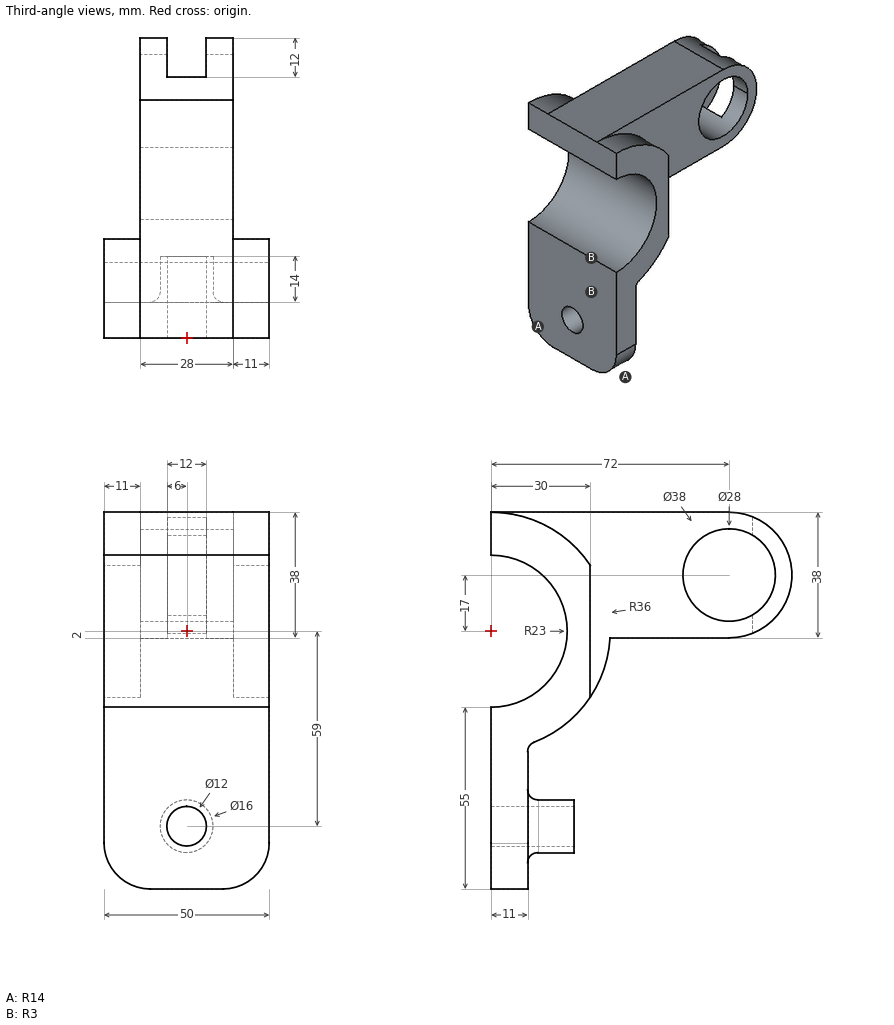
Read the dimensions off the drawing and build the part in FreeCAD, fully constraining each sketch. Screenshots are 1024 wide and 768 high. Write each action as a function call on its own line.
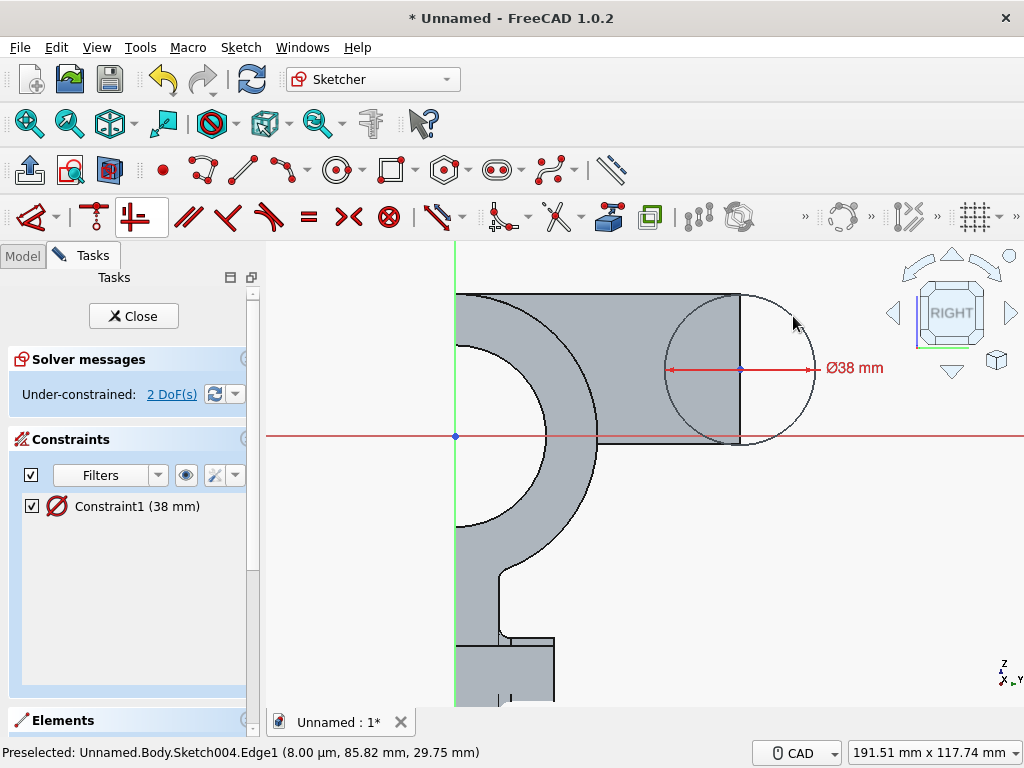
click(32, 218)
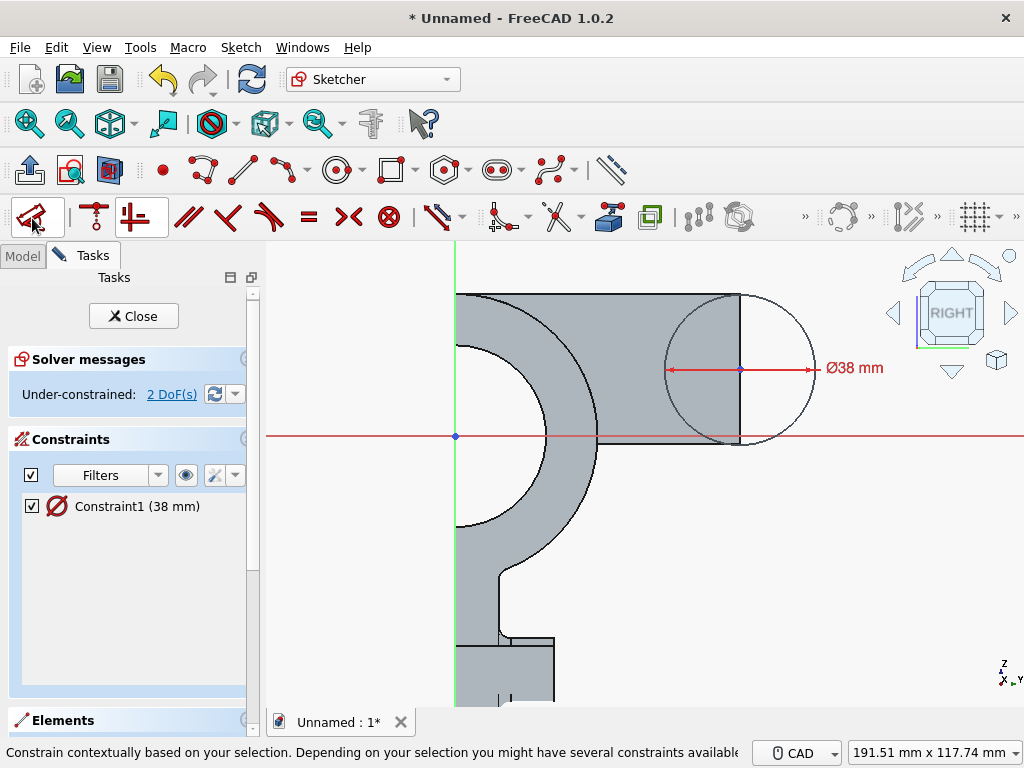
click(740, 370)
click(598, 470)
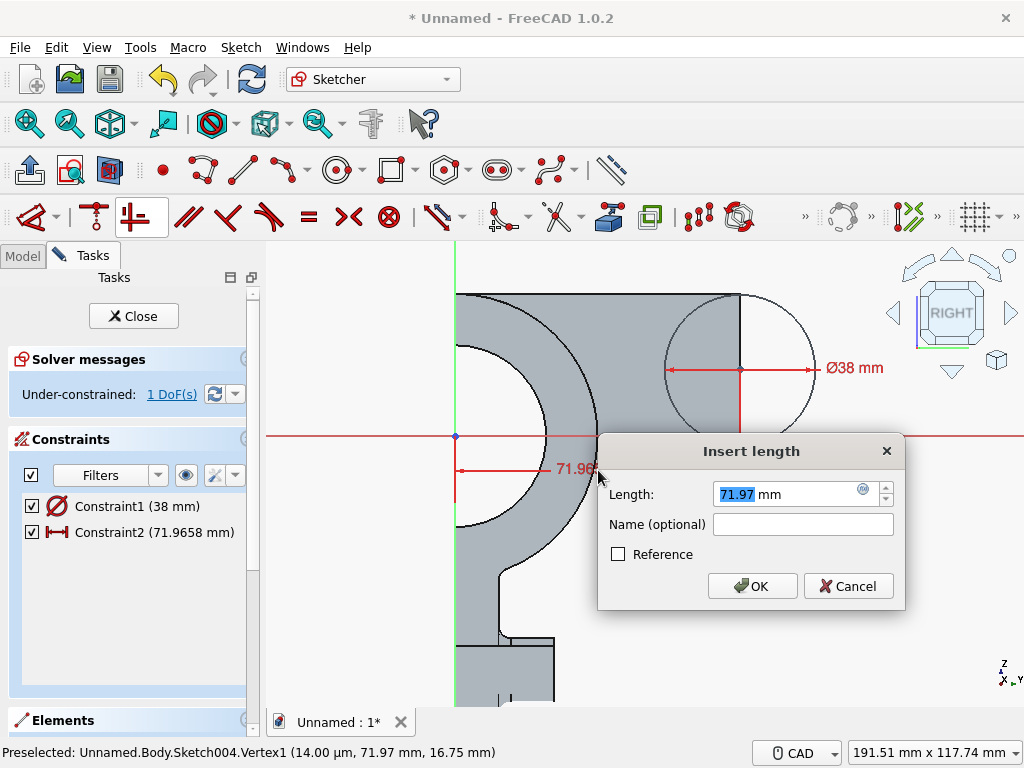
text(72)
key(Return)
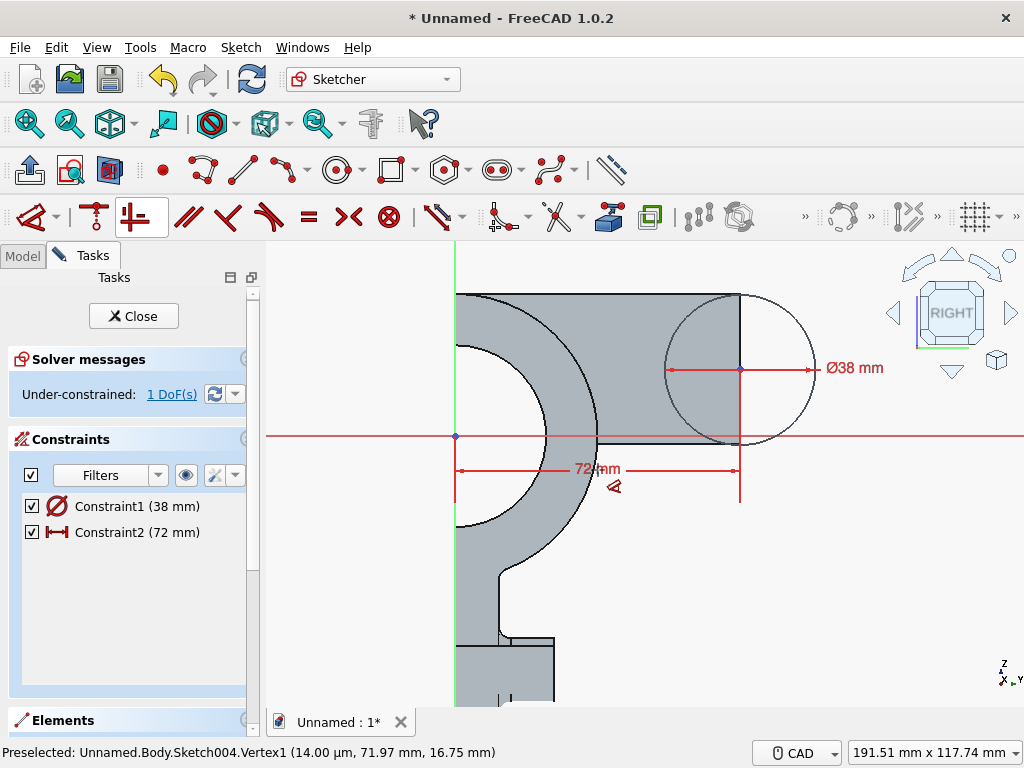
click(740, 370)
click(421, 403)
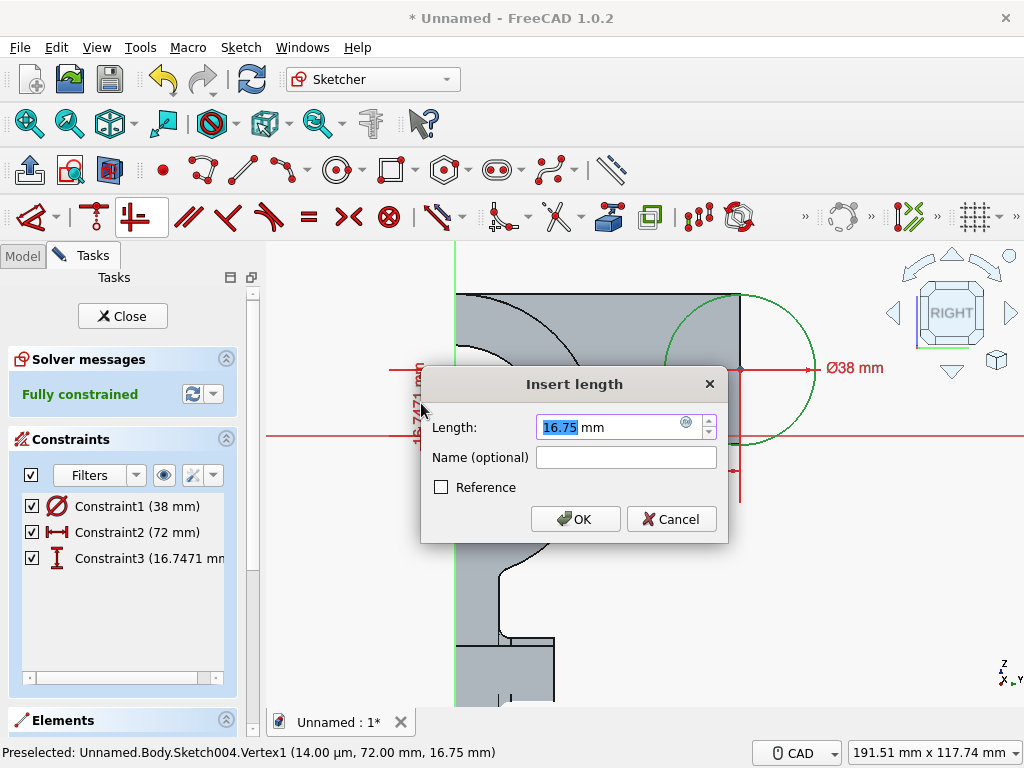
text(17)
key(Return)
key(Escape)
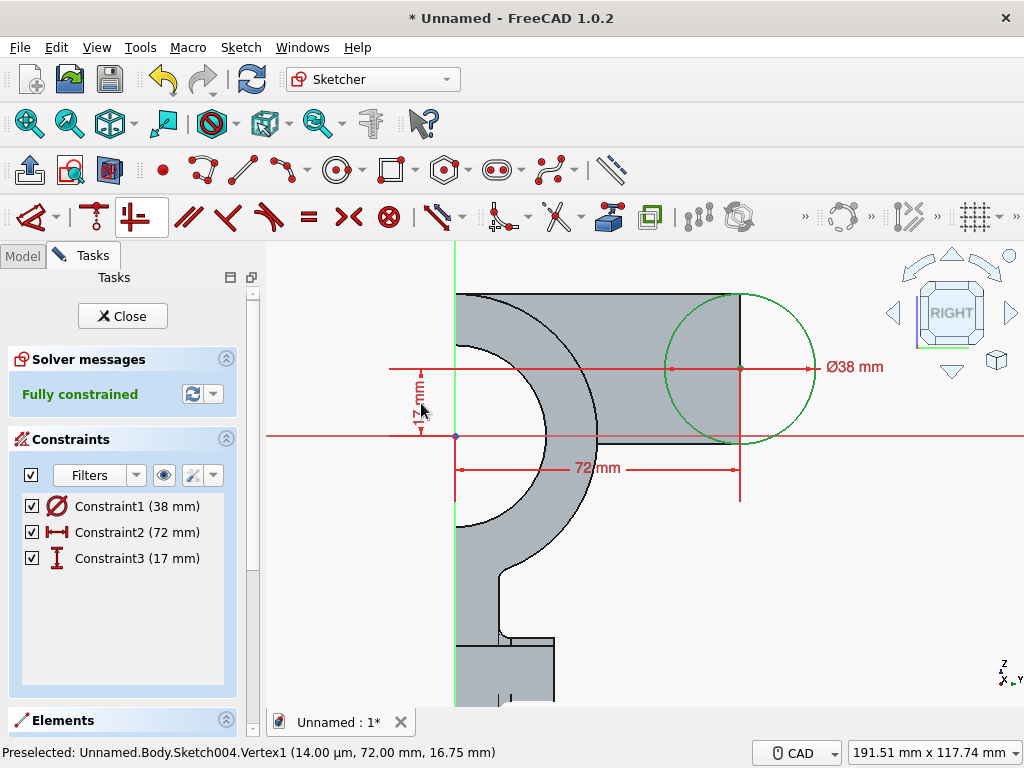
click(123, 316)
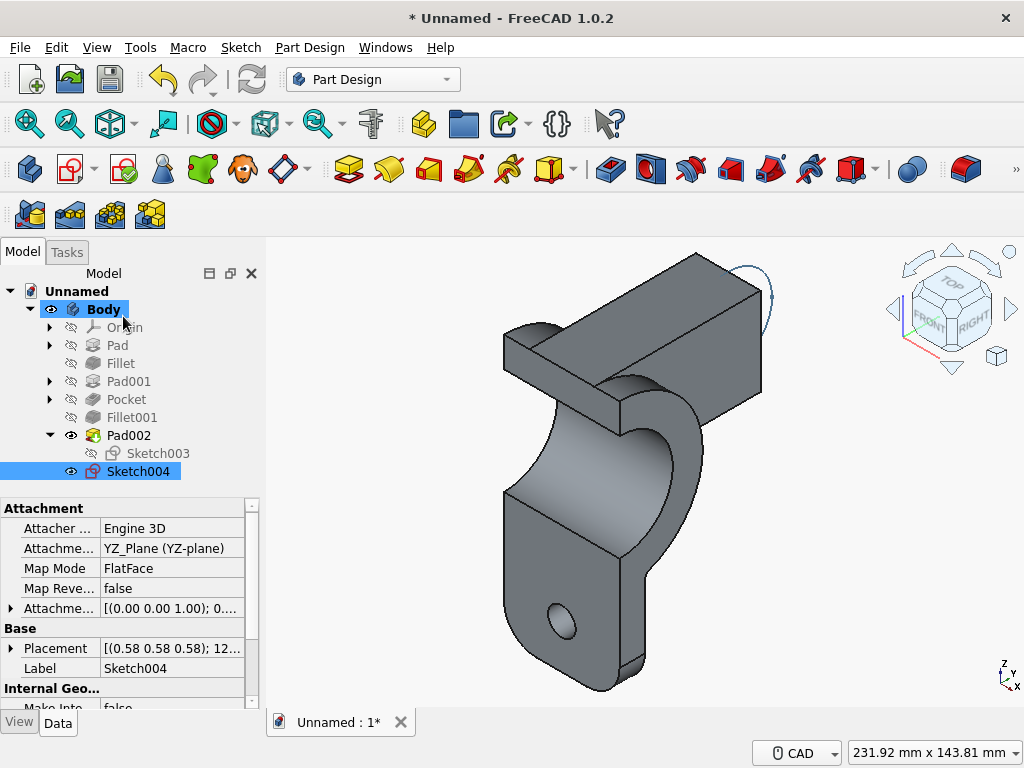
click(350, 170)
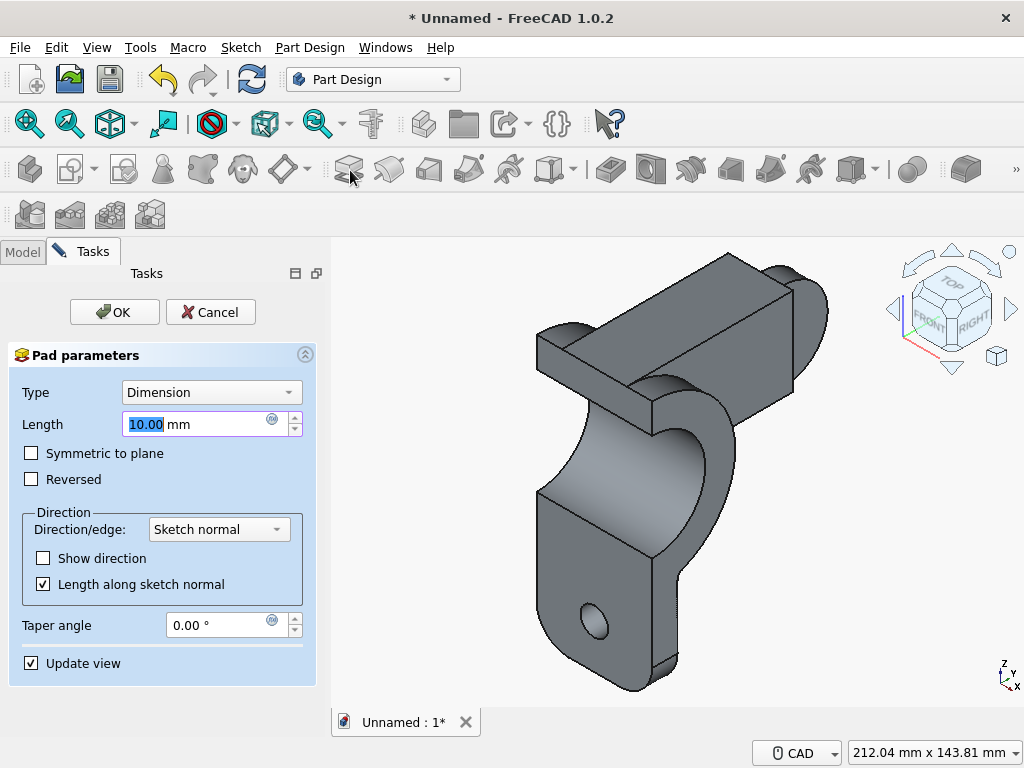
text(28)
key(Tab)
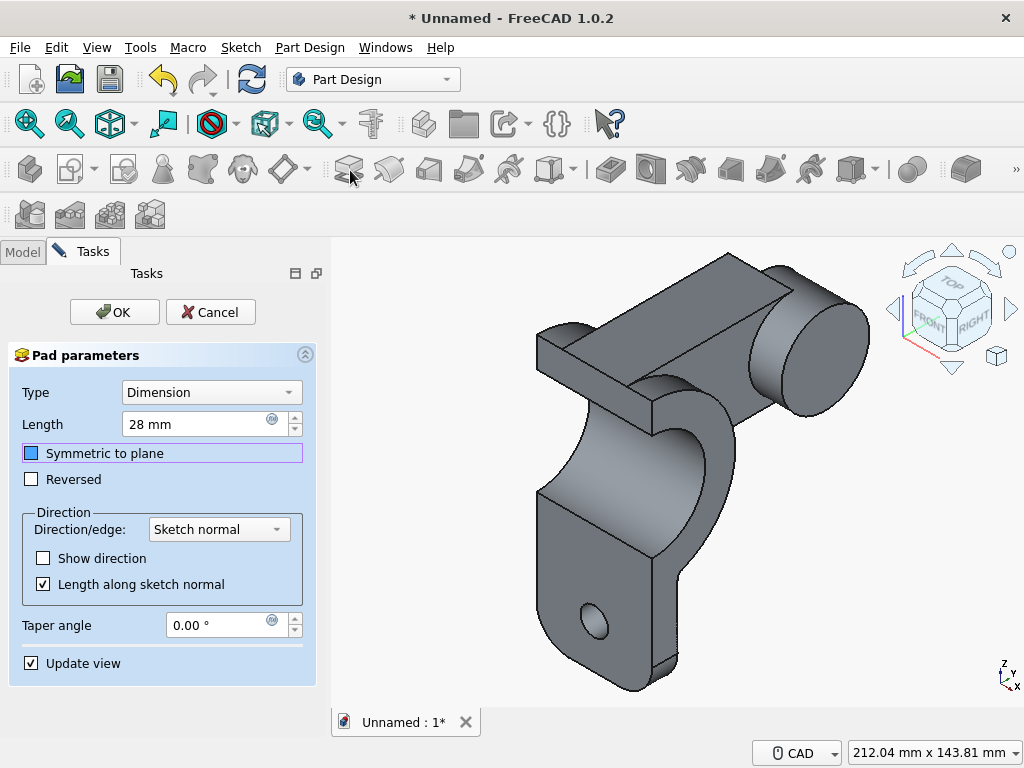
click(30, 453)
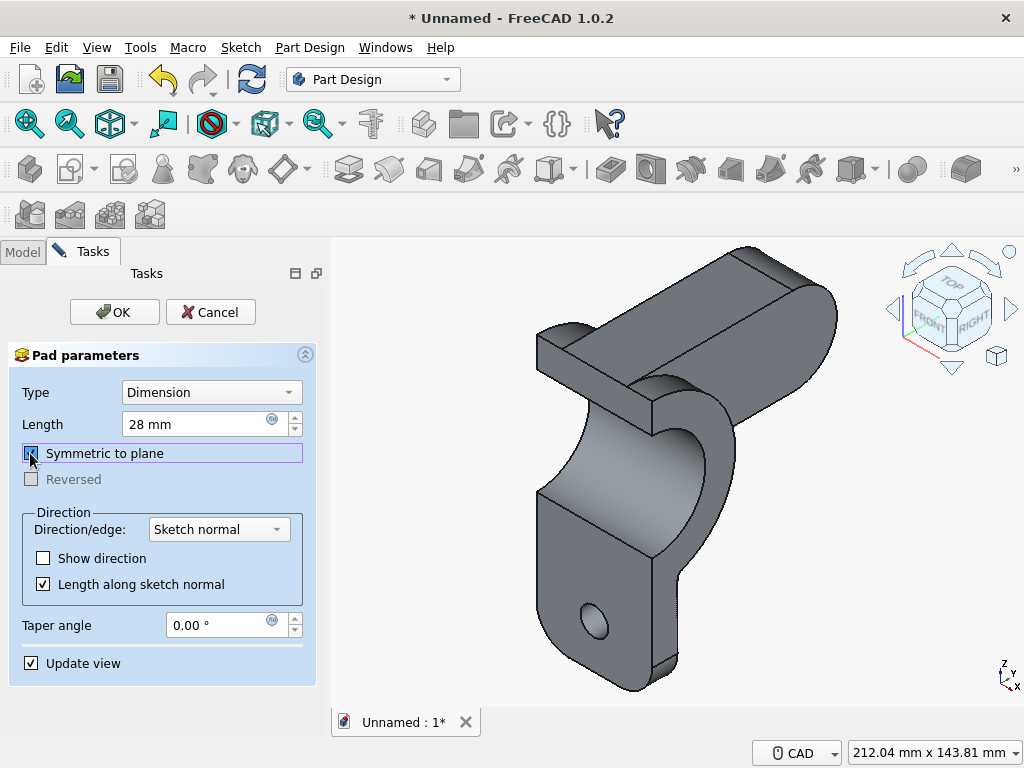
click(115, 312)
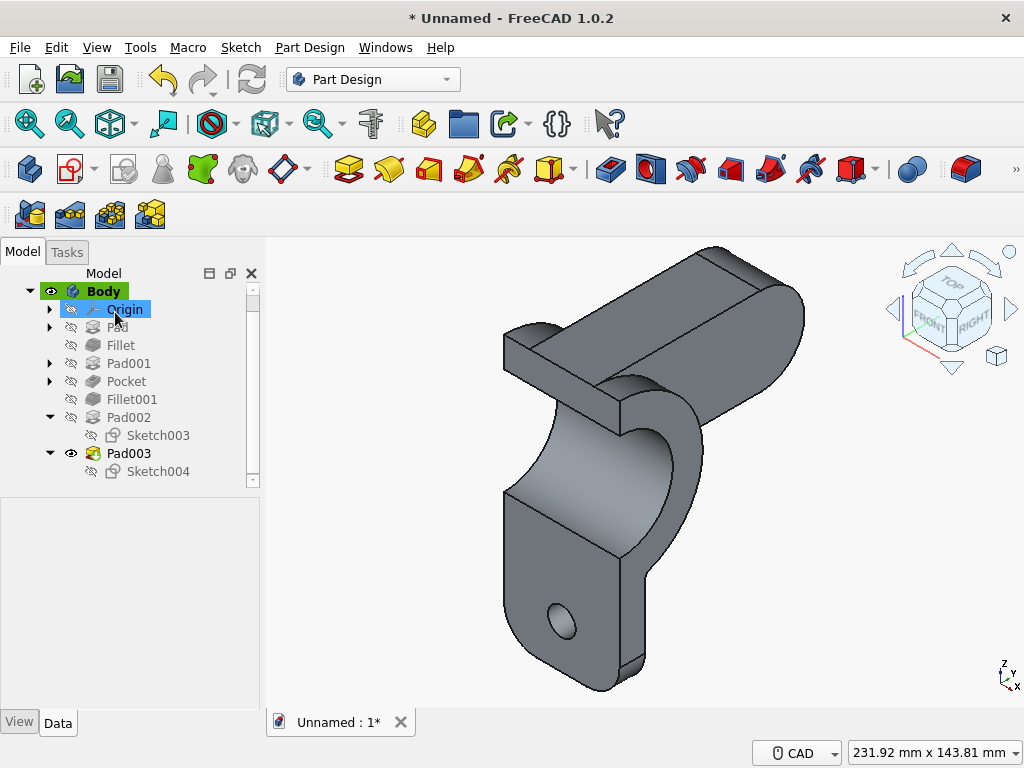
click(30, 124)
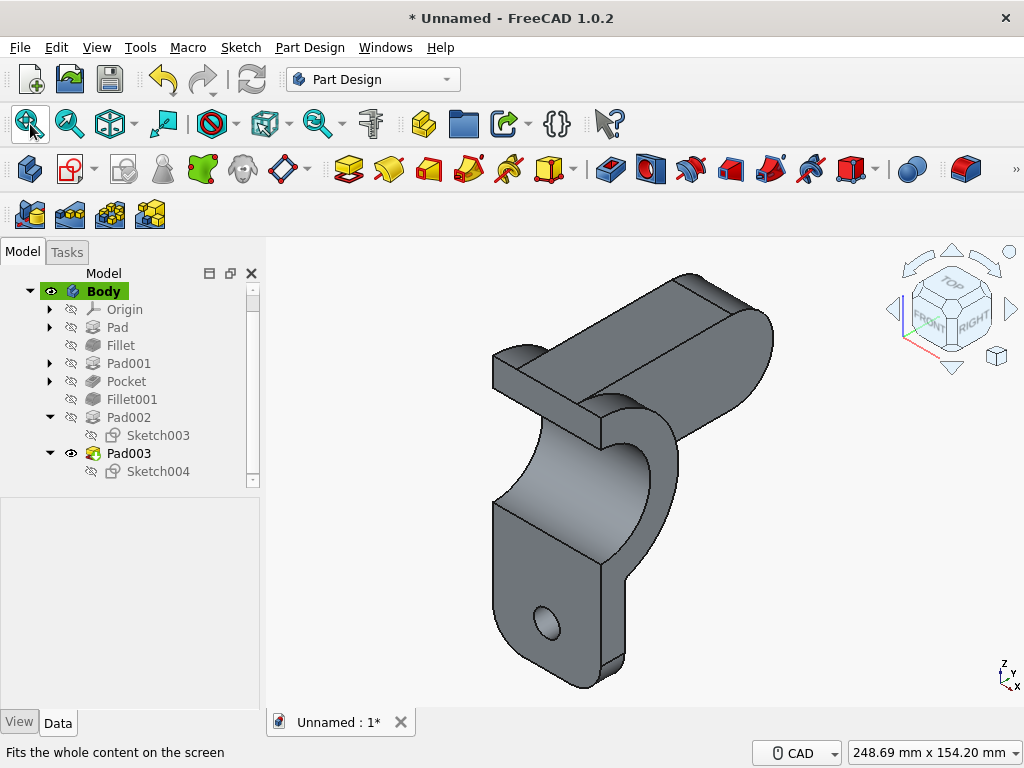
key(6)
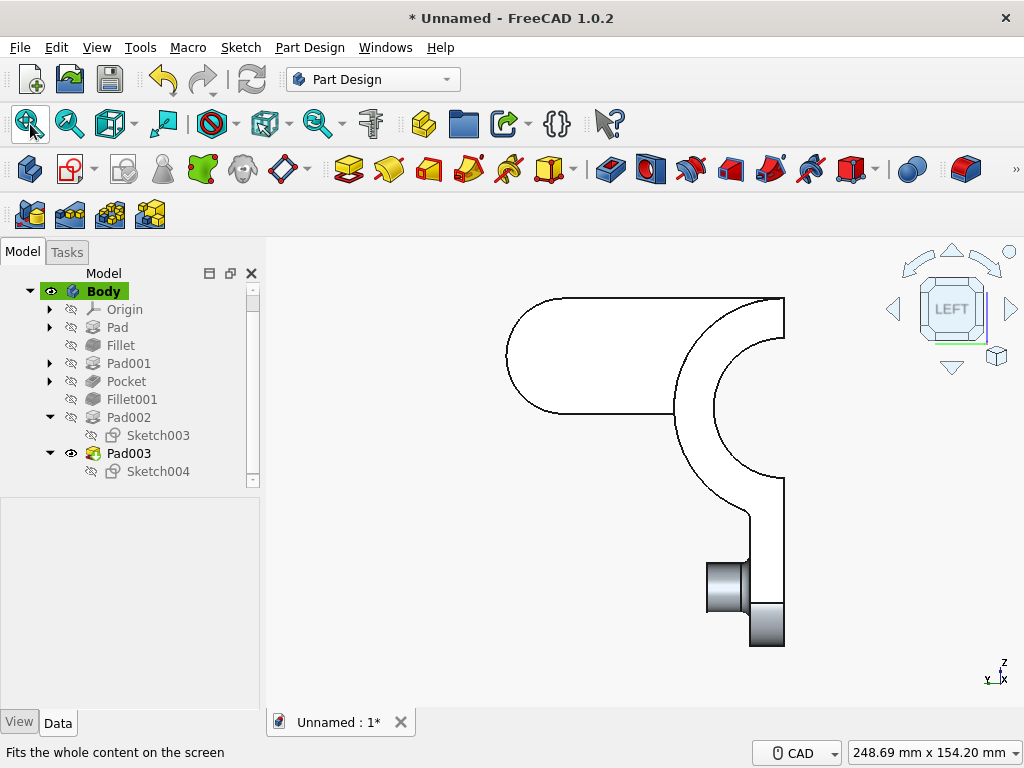
click(605, 355)